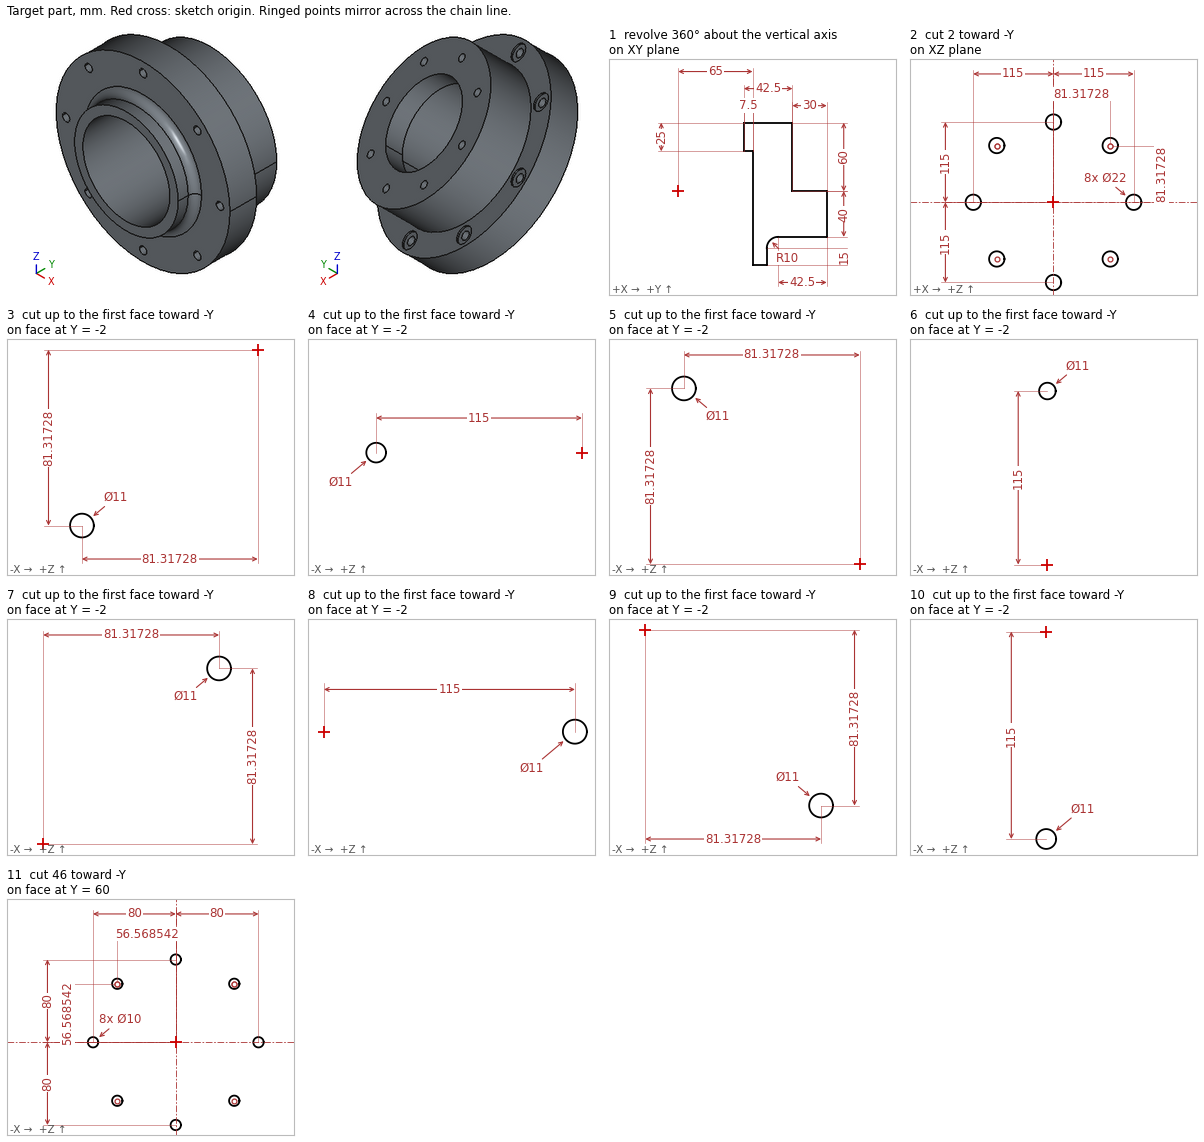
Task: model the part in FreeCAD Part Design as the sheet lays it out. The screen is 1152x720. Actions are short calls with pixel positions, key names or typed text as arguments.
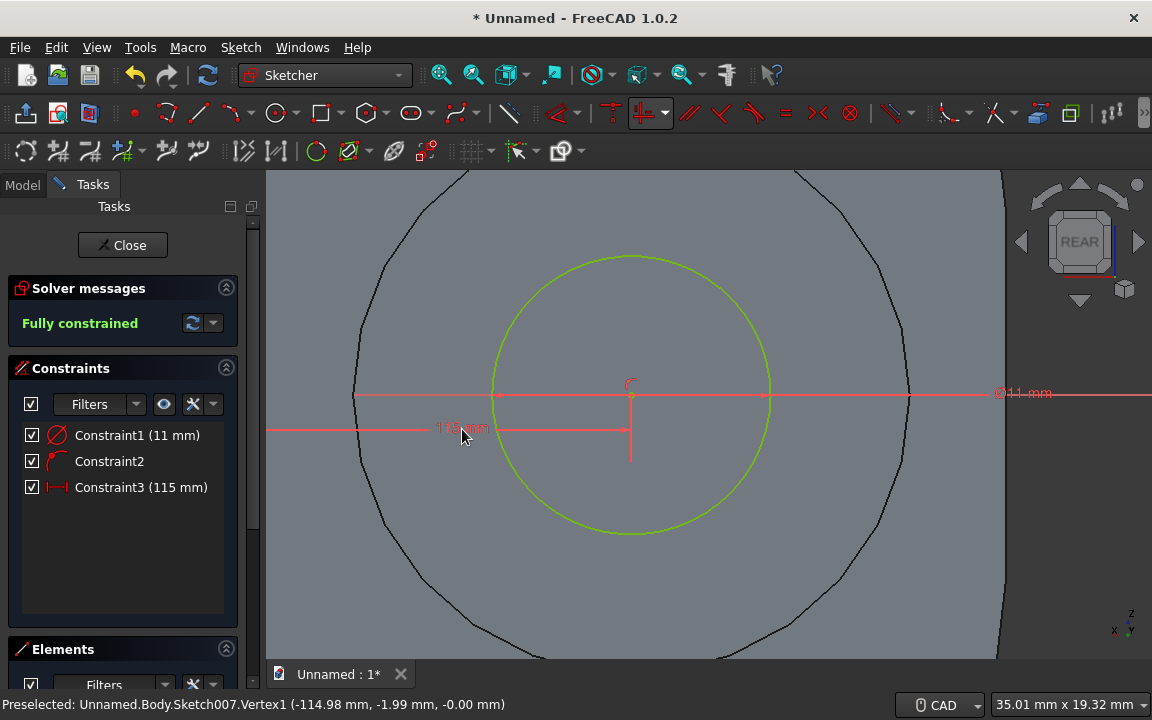
click(123, 245)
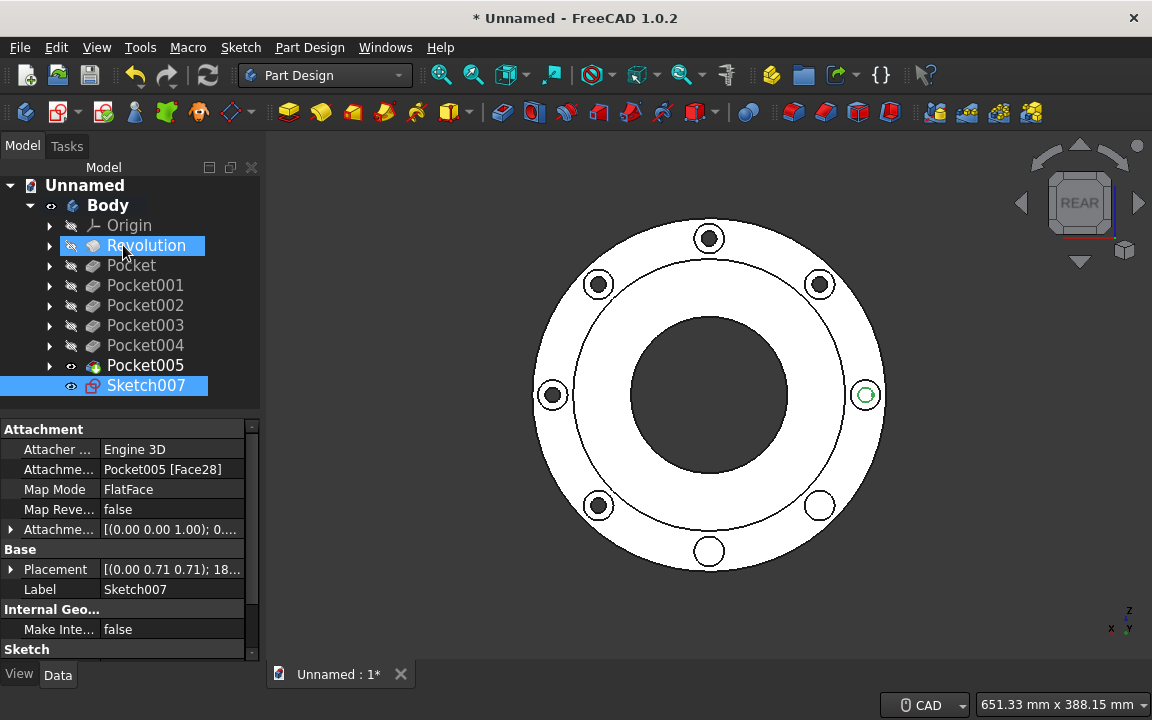
click(504, 112)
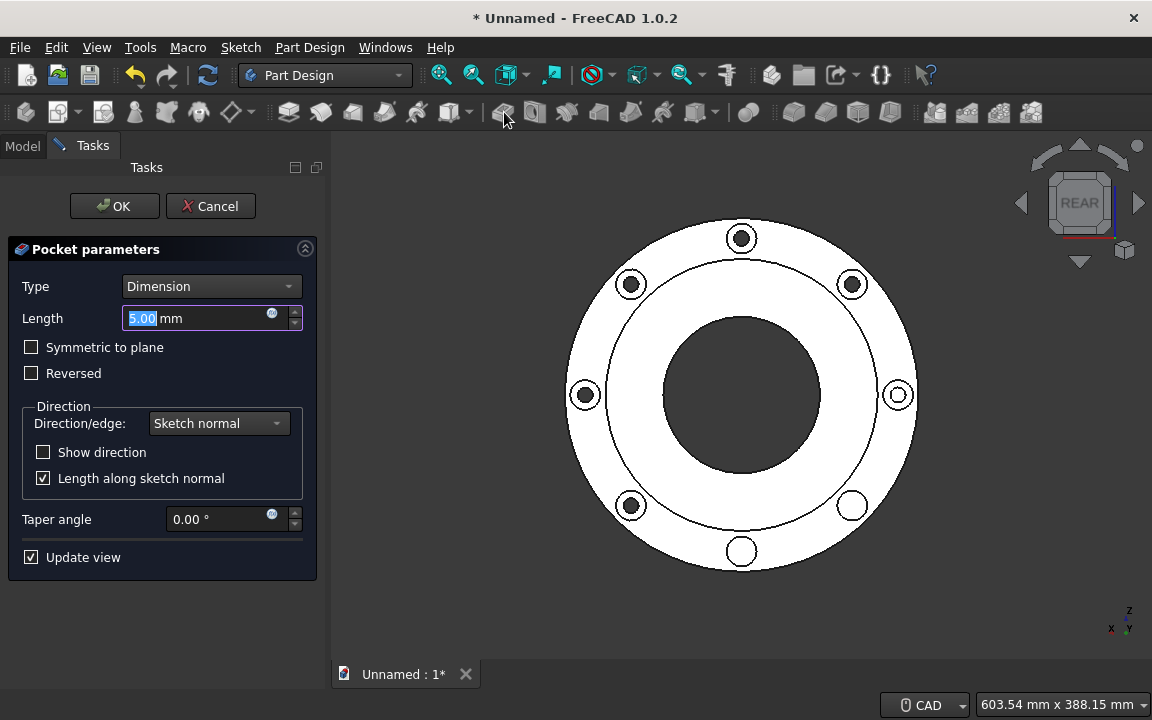
click(212, 286)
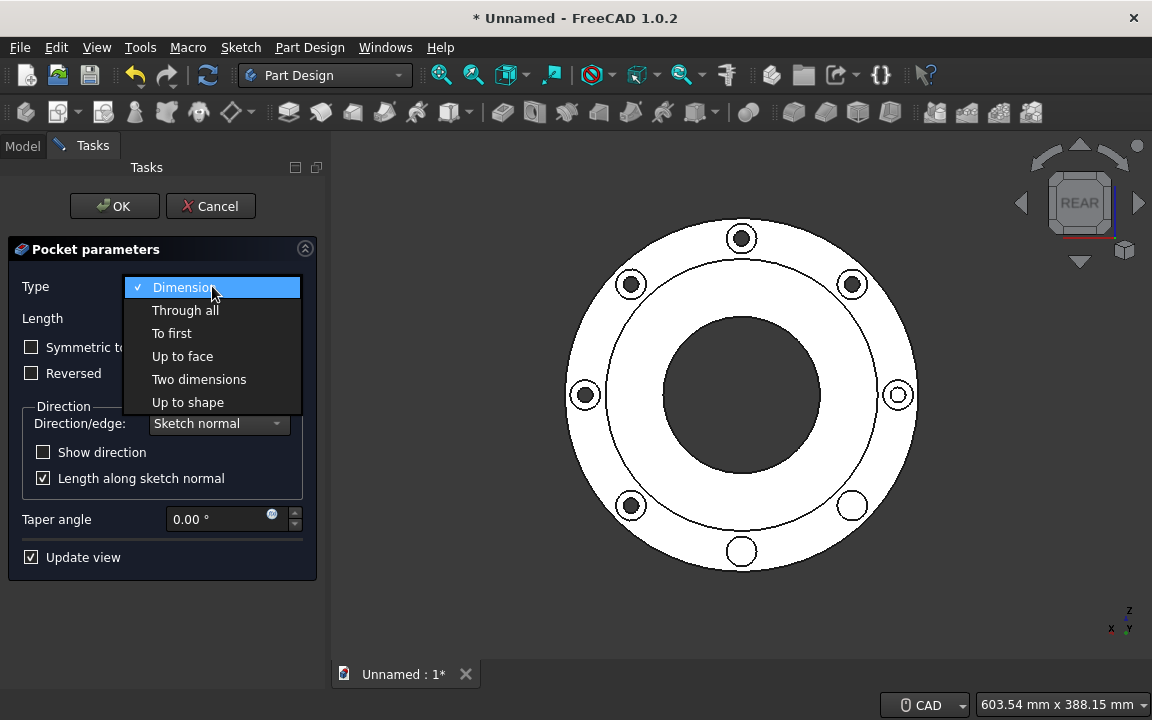
click(212, 334)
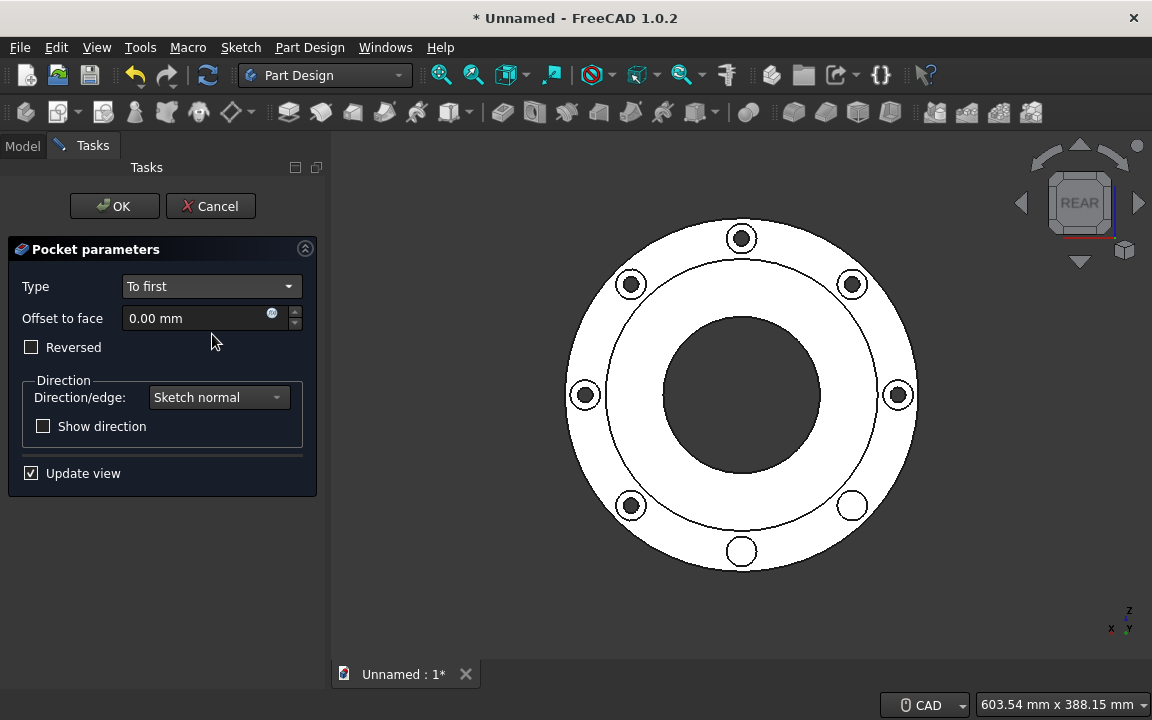
click(115, 206)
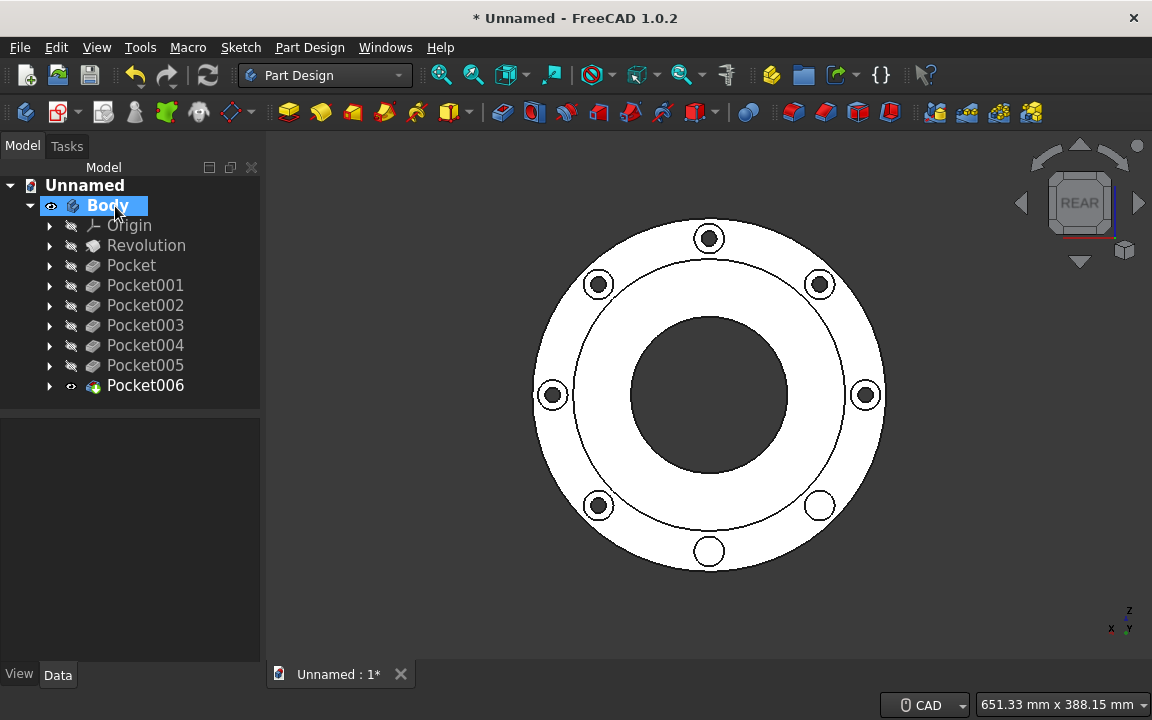
click(709, 550)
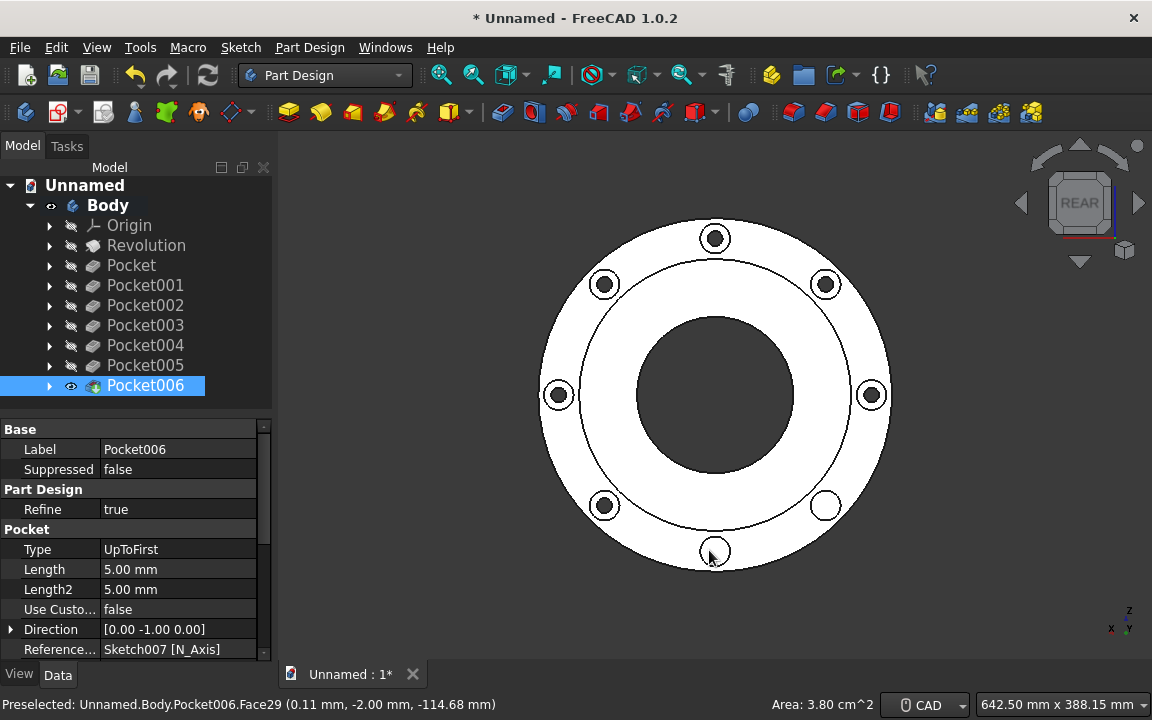
click(58, 112)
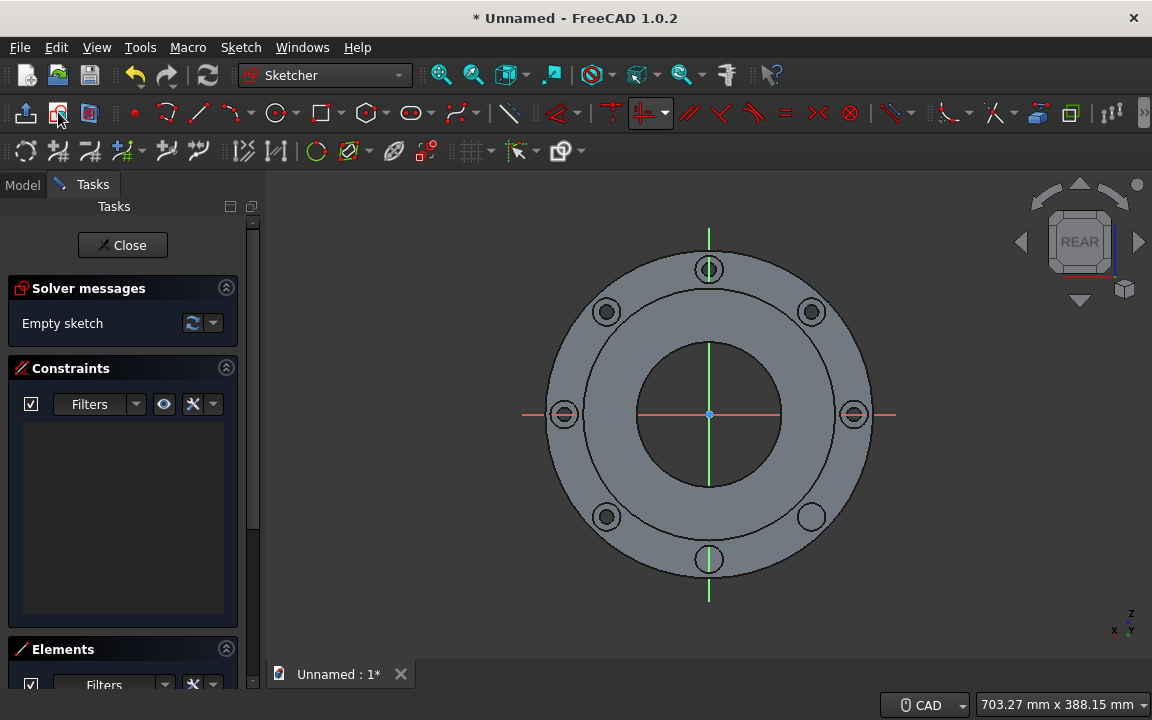
click(90, 114)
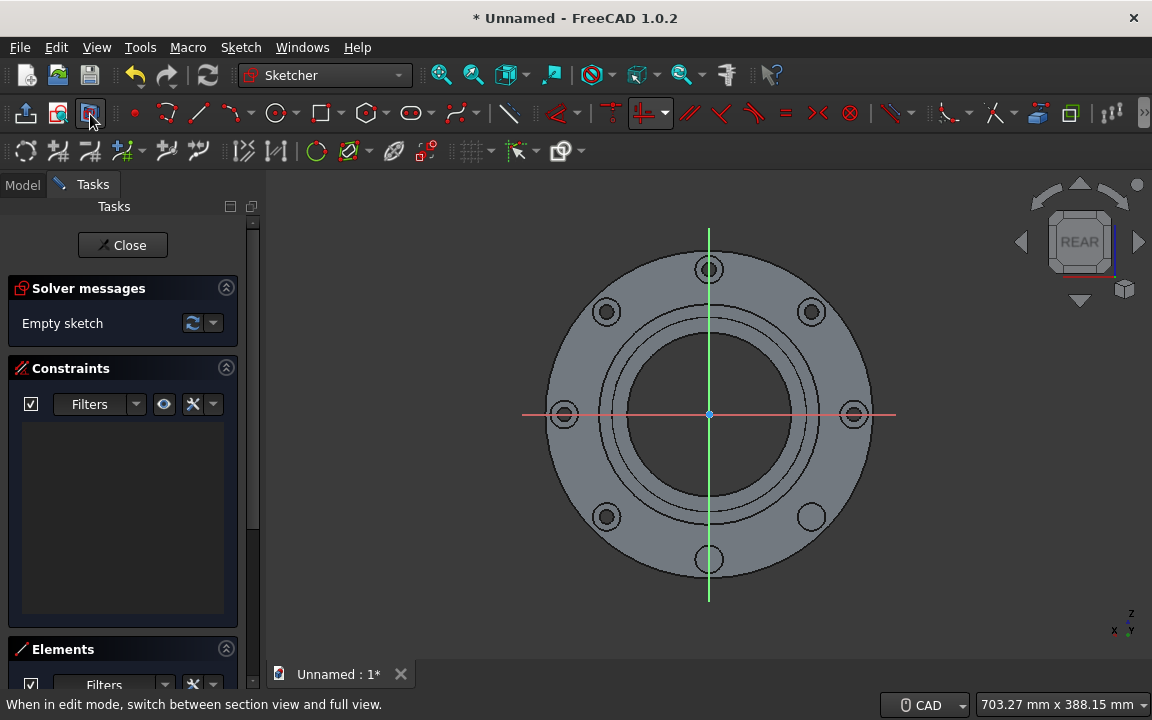
scroll(821, 522, up, 15)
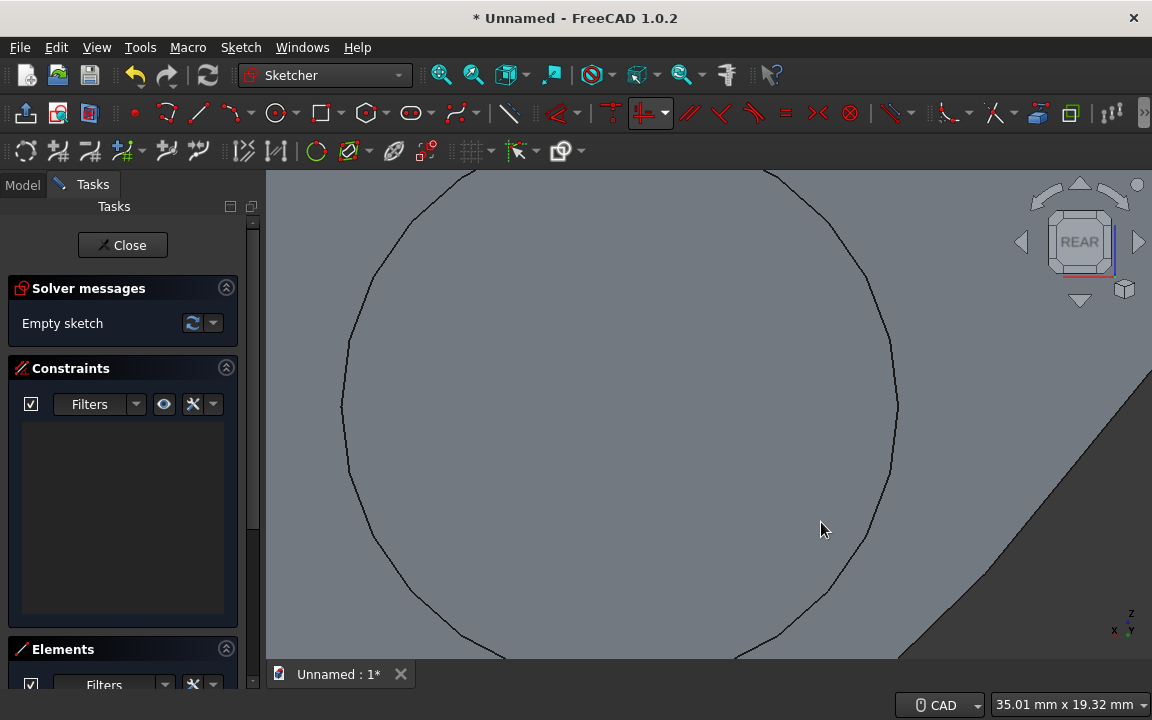
key(g)
key(c)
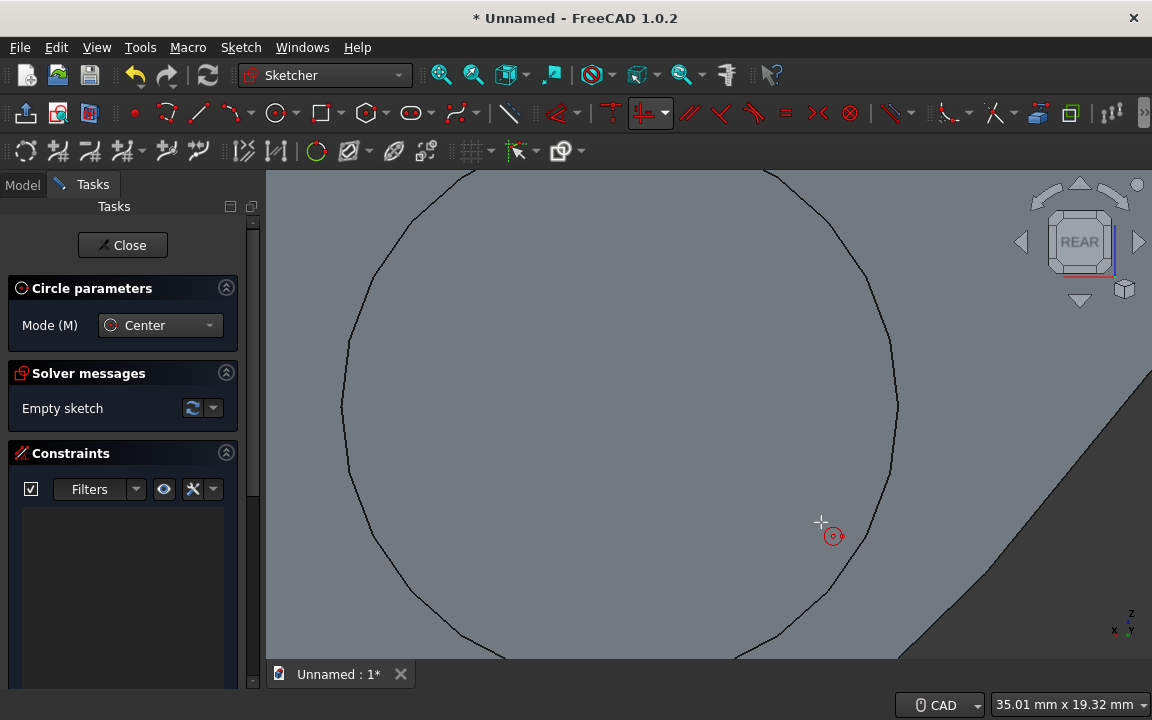
click(620, 407)
move(718, 308)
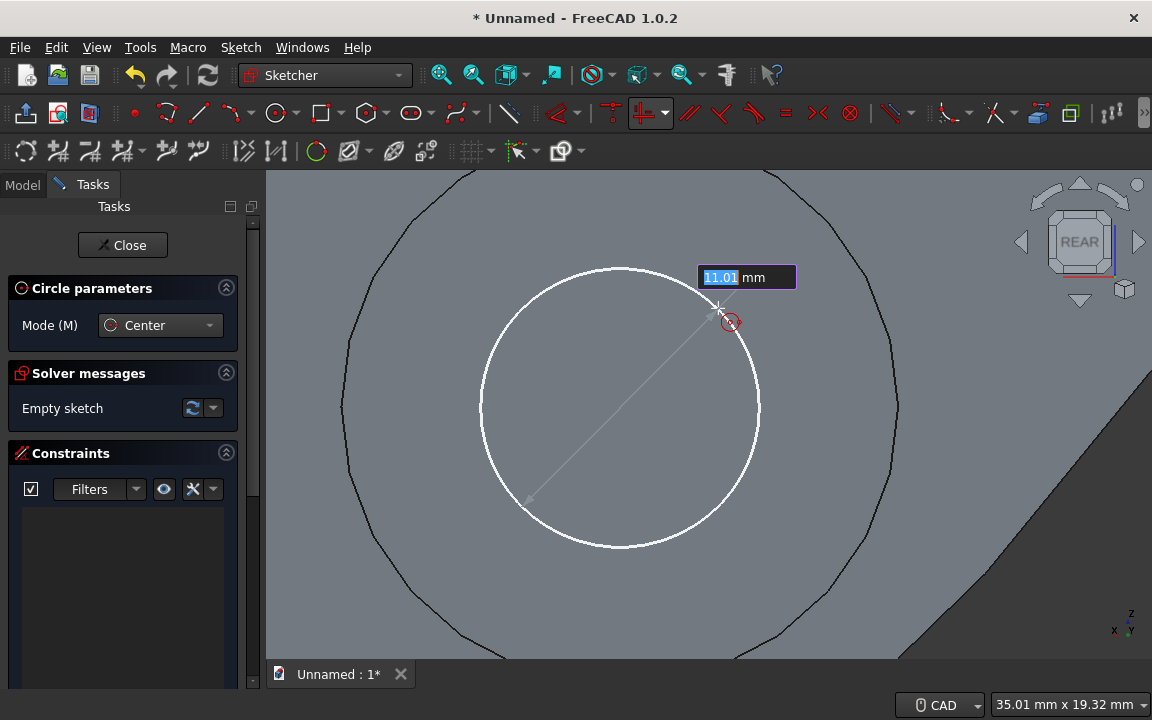
text(11)
key(Return)
key(Escape)